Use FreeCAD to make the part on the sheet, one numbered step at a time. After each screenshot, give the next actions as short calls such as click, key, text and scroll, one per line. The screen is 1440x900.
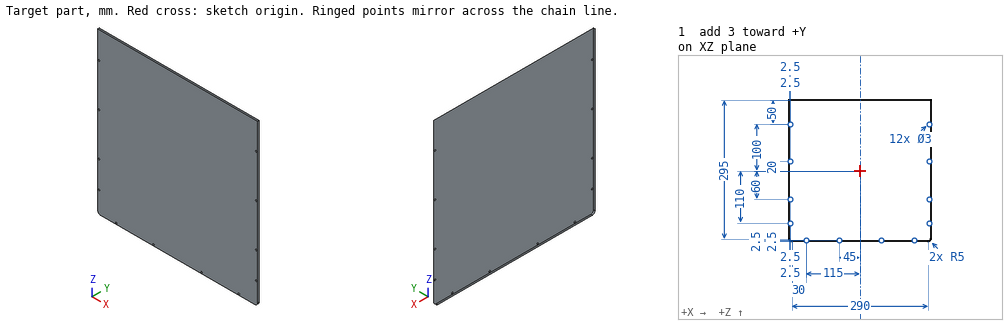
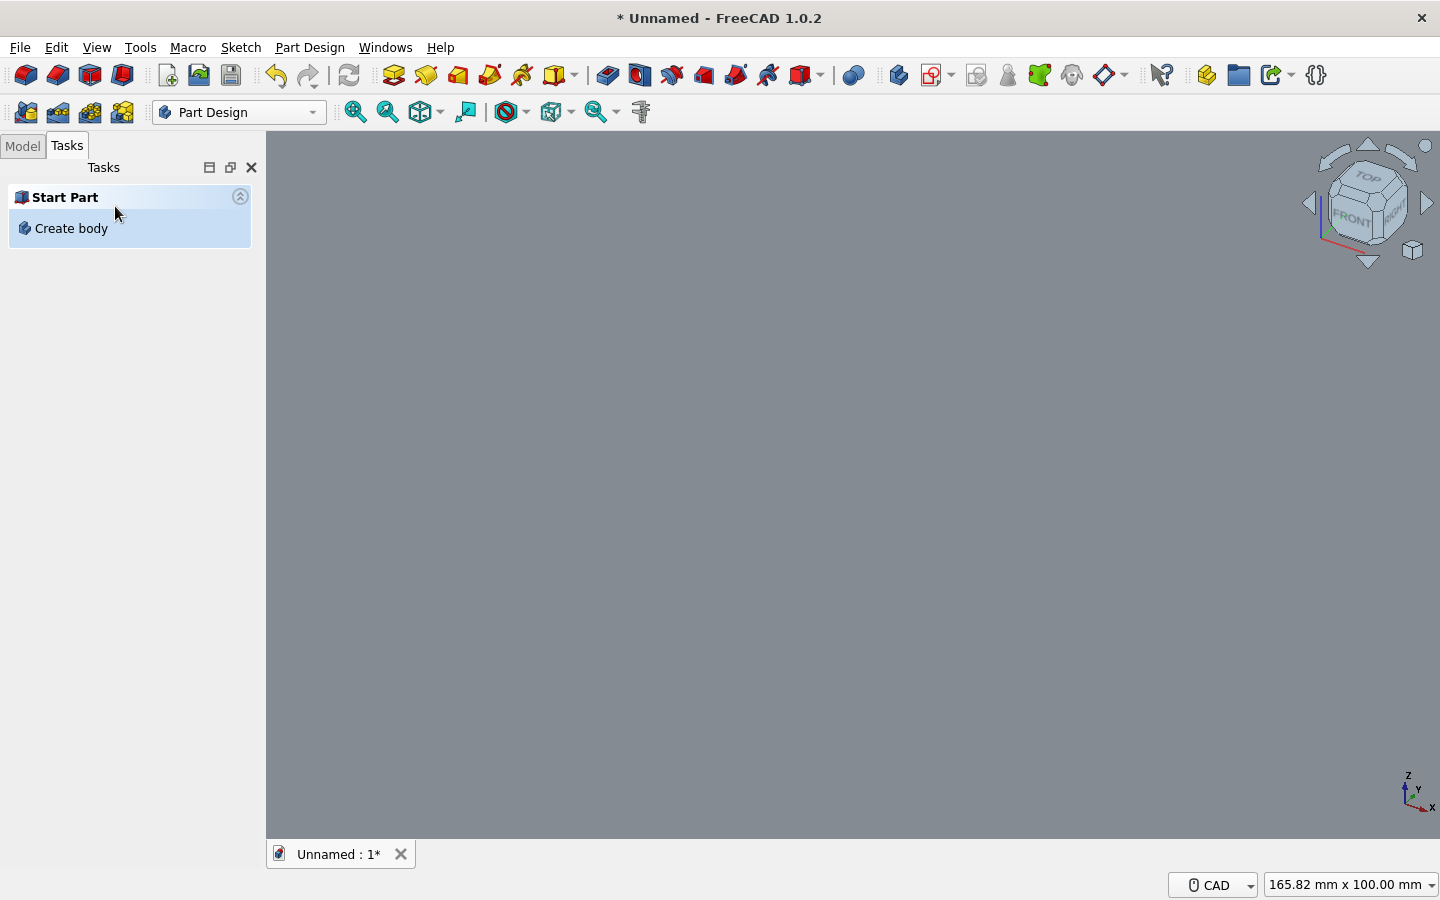
key(0)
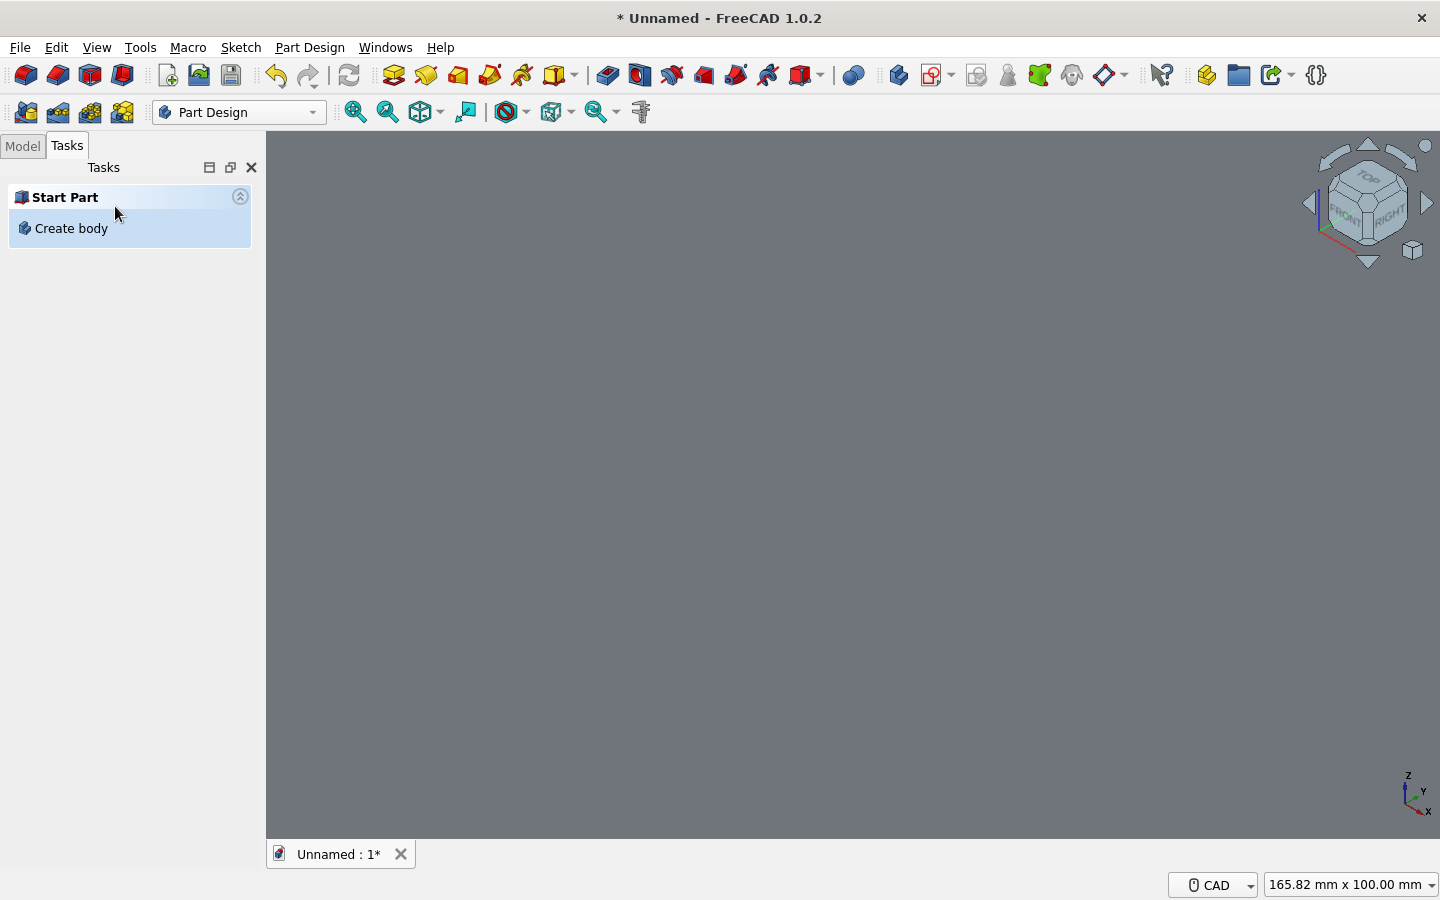
click(356, 112)